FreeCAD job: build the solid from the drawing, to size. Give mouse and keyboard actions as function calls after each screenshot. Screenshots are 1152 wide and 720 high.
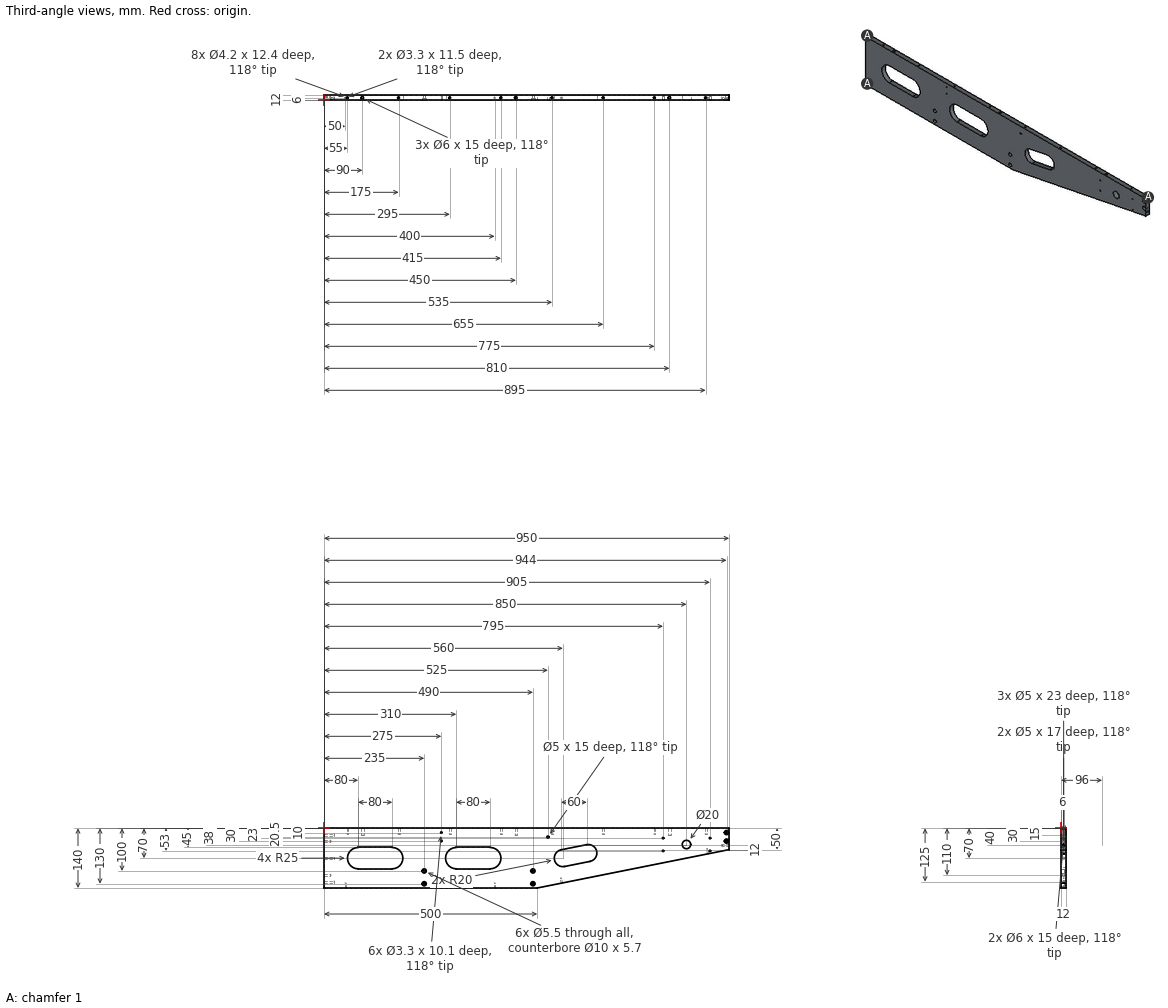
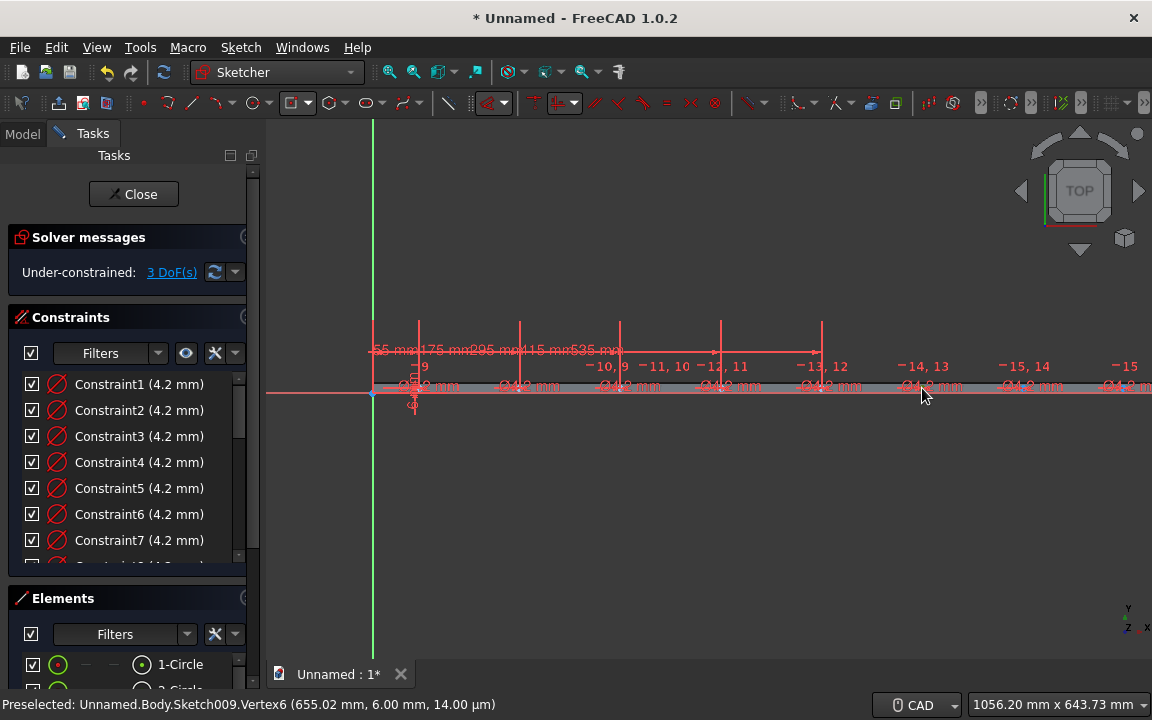
key(l)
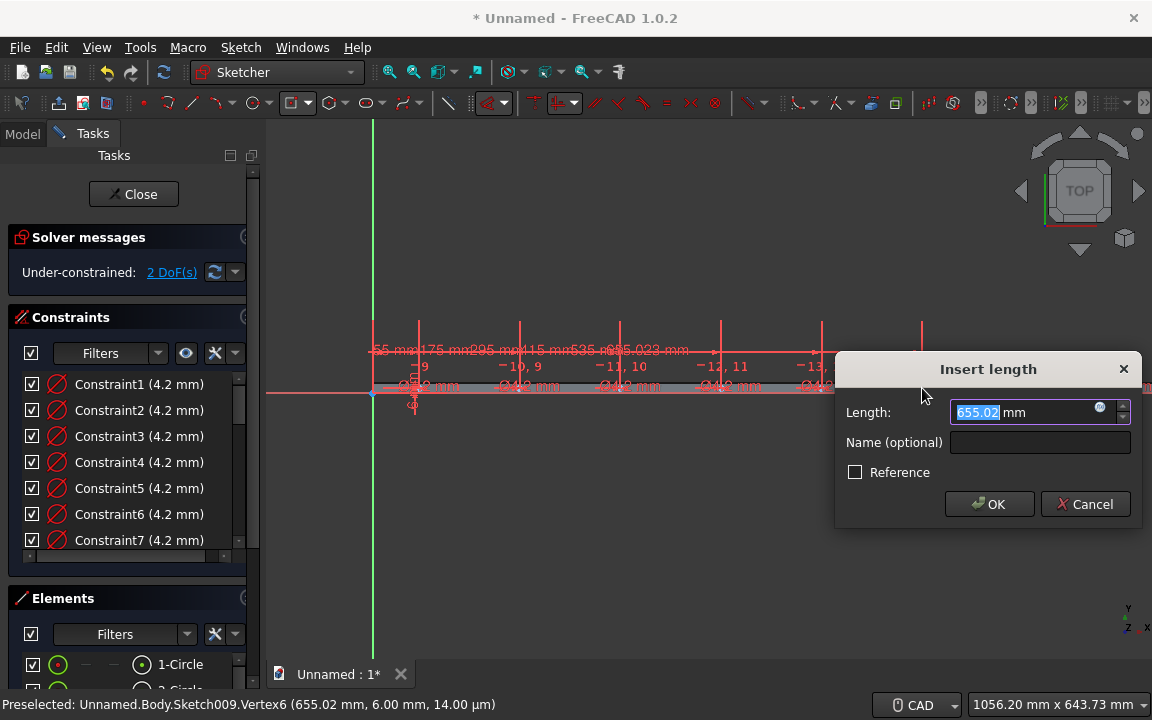
text(655)
key(Return)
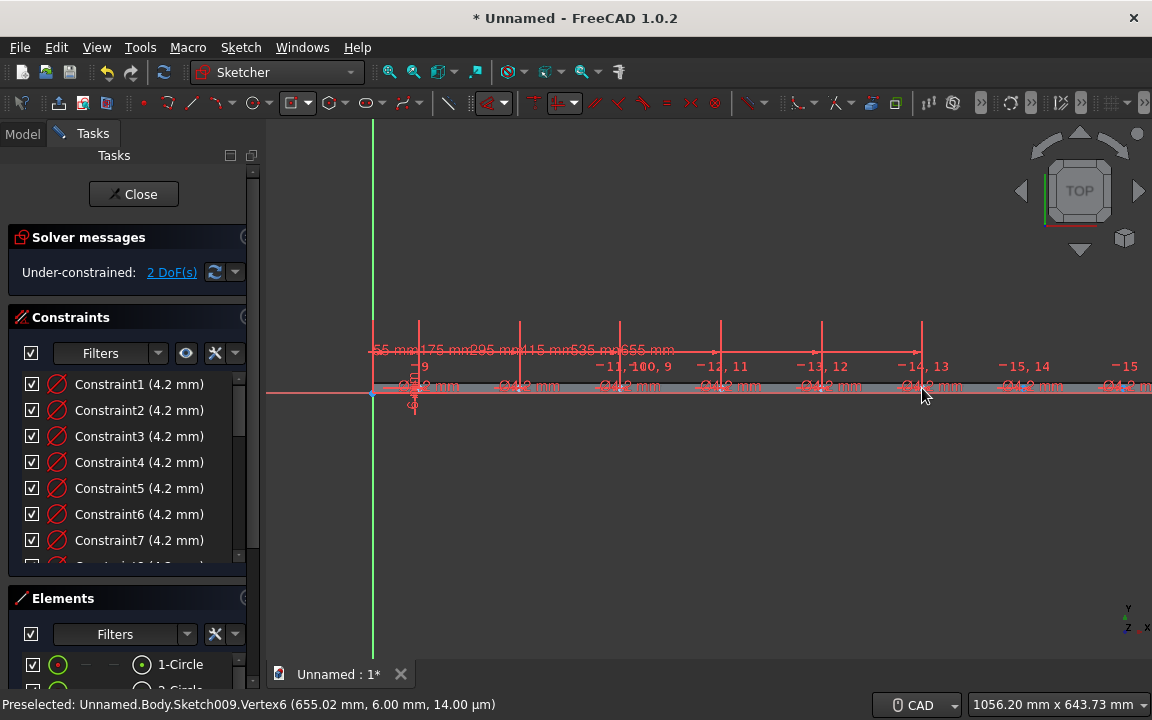
scroll(419, 387, down, 2)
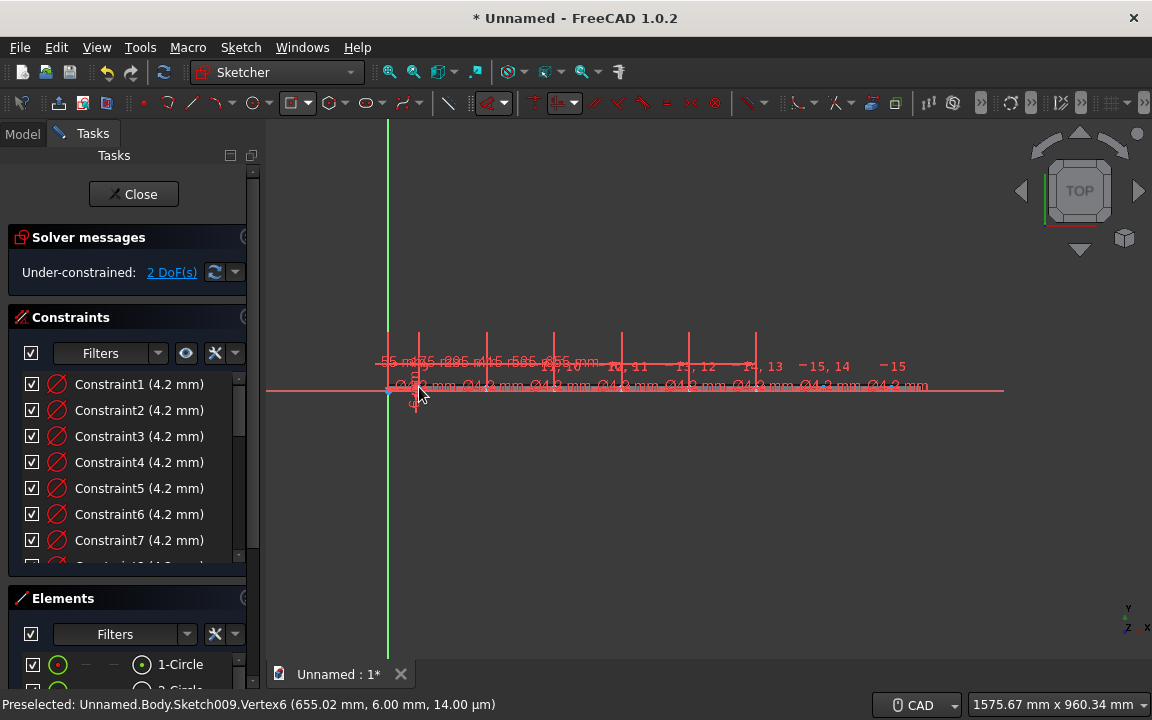
click(824, 388)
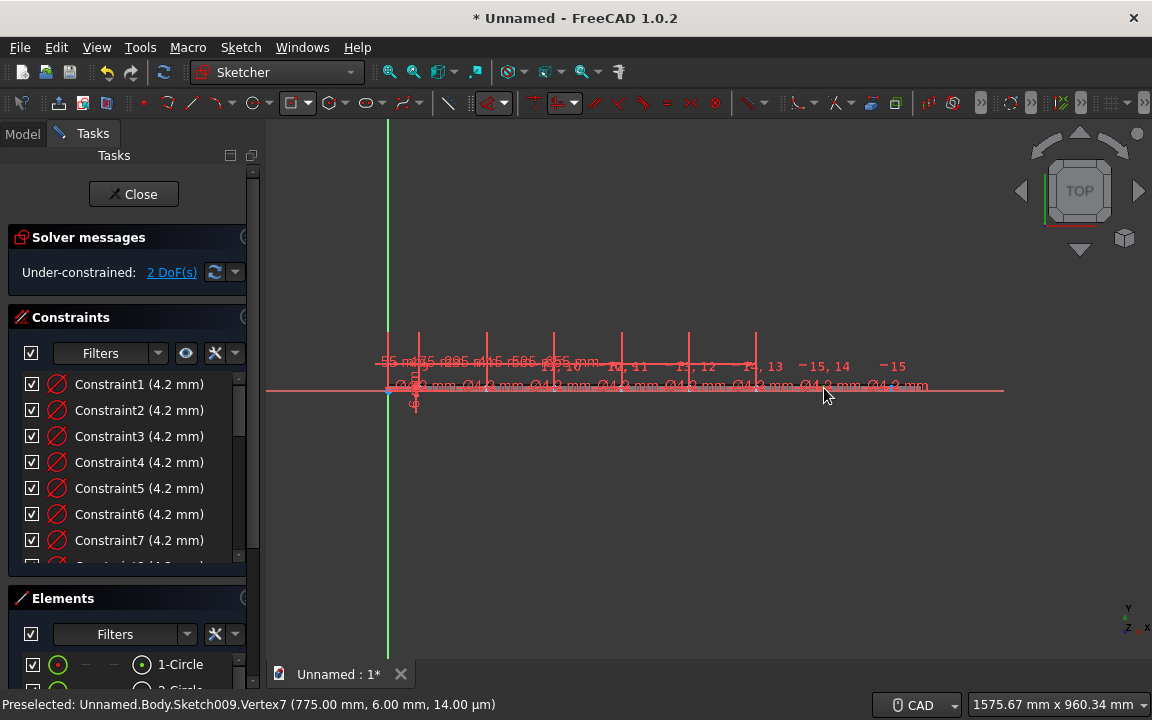
key(l)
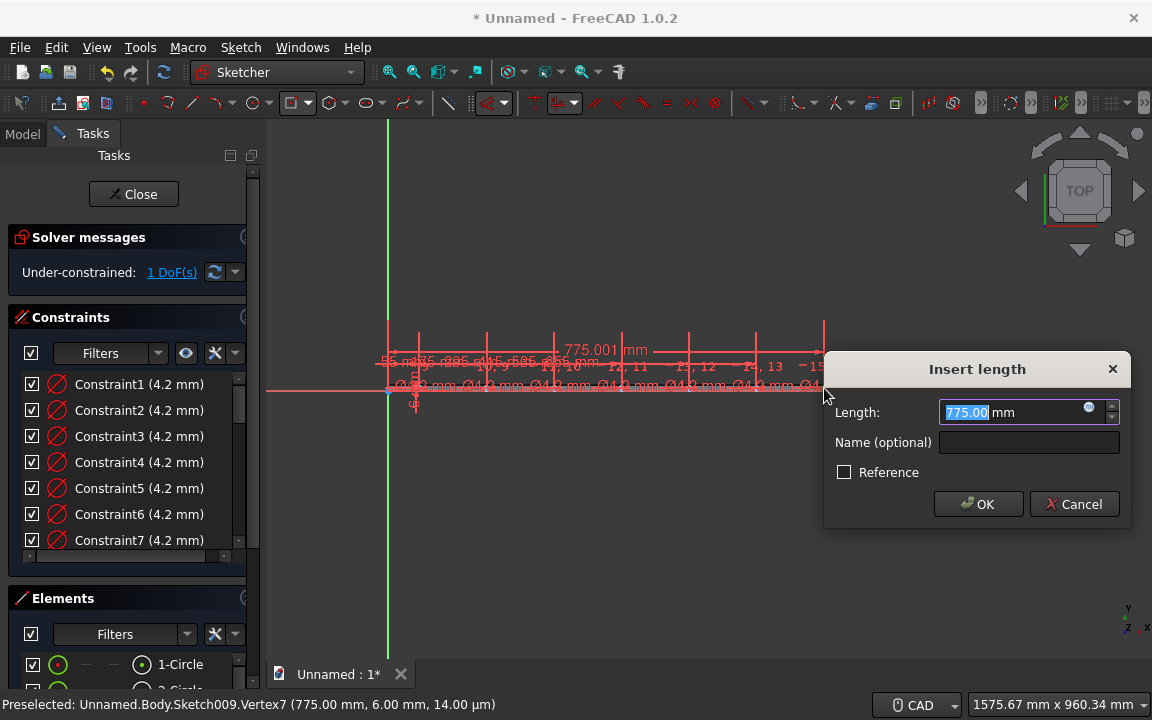
text(775)
key(Return)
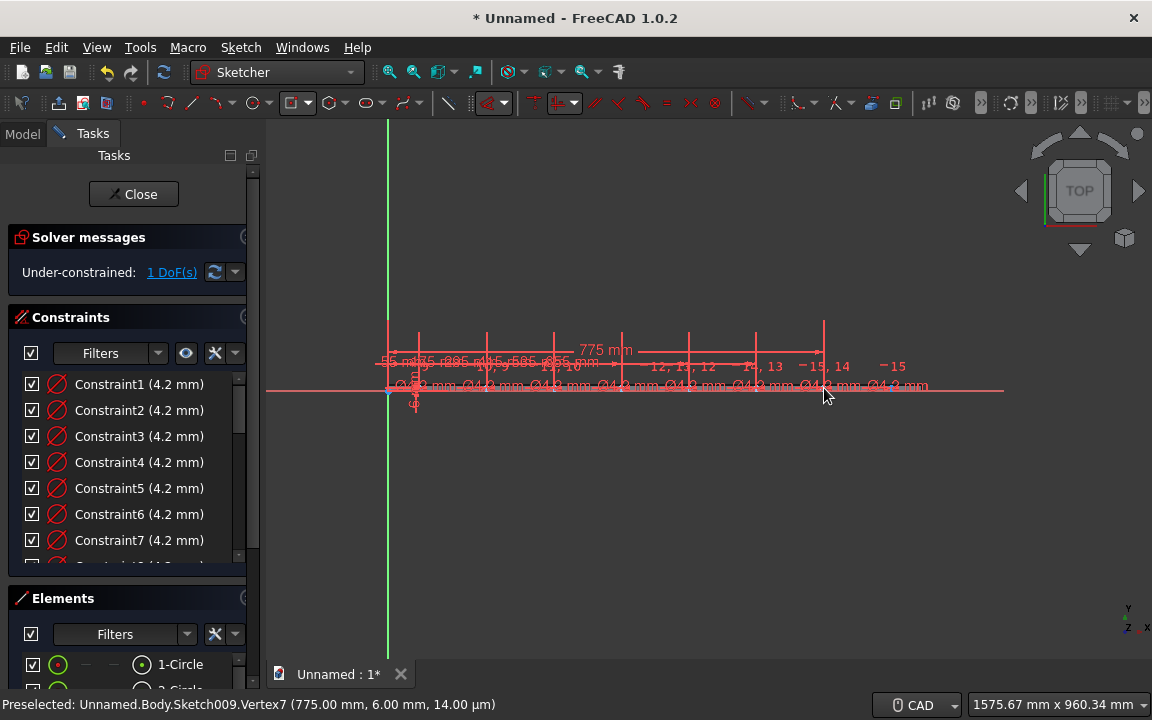
click(891, 388)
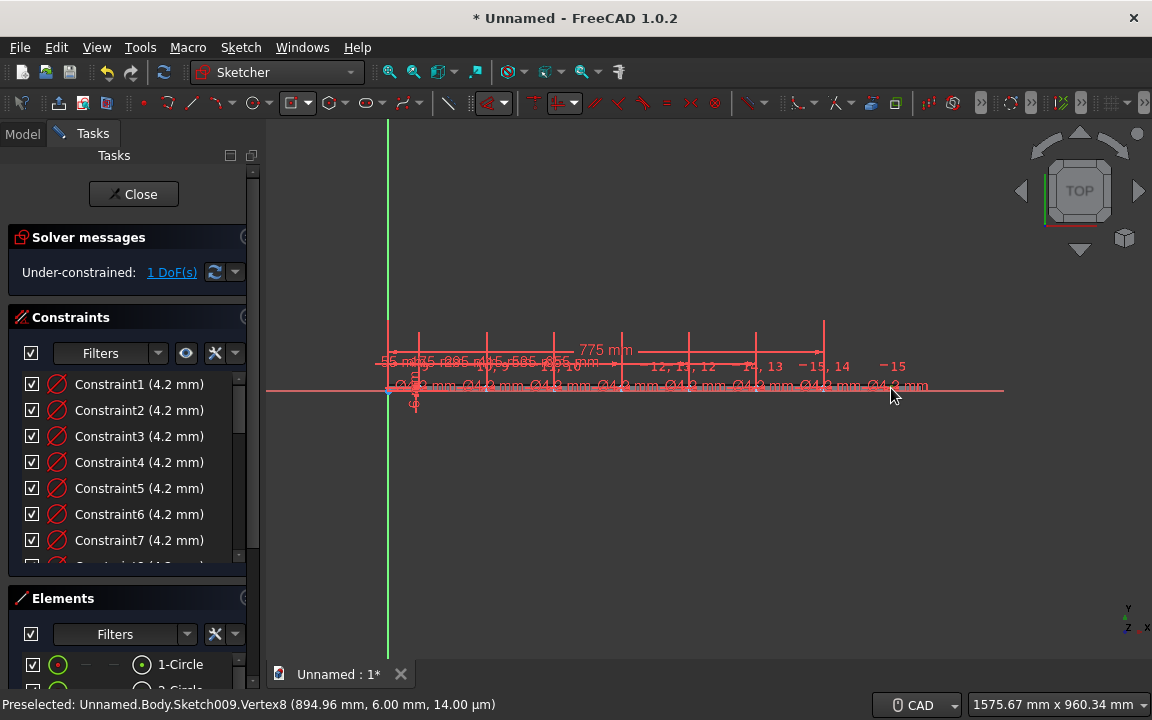
key(l)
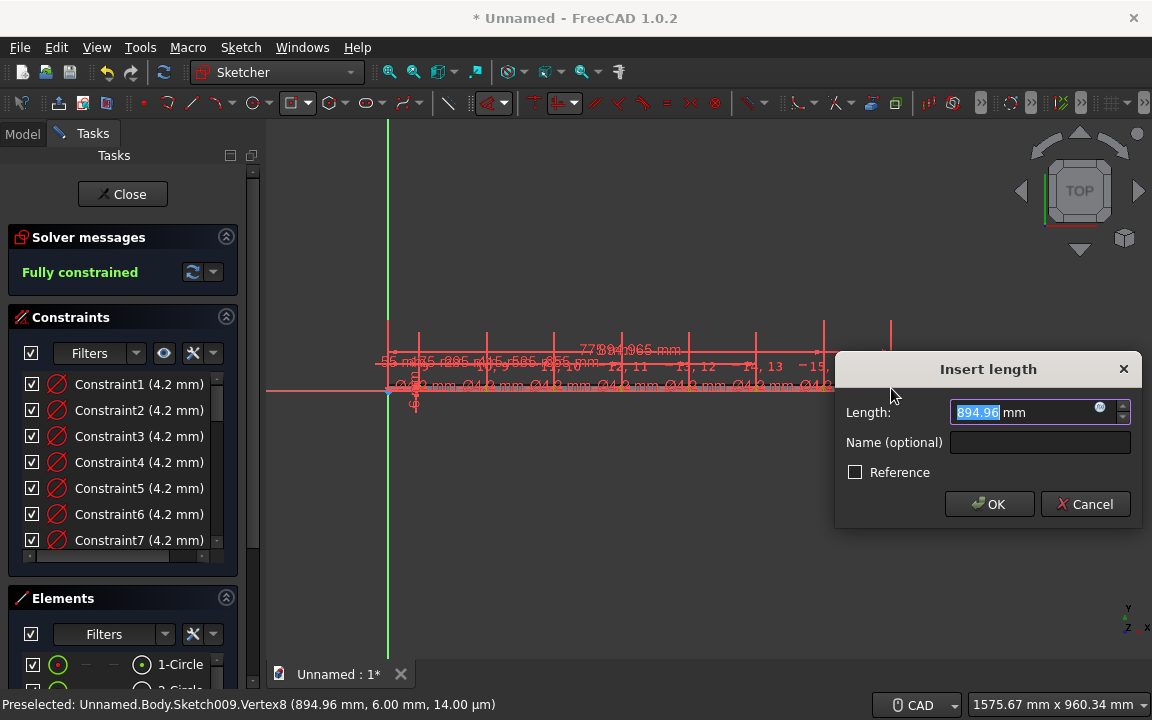
text(895)
key(Return)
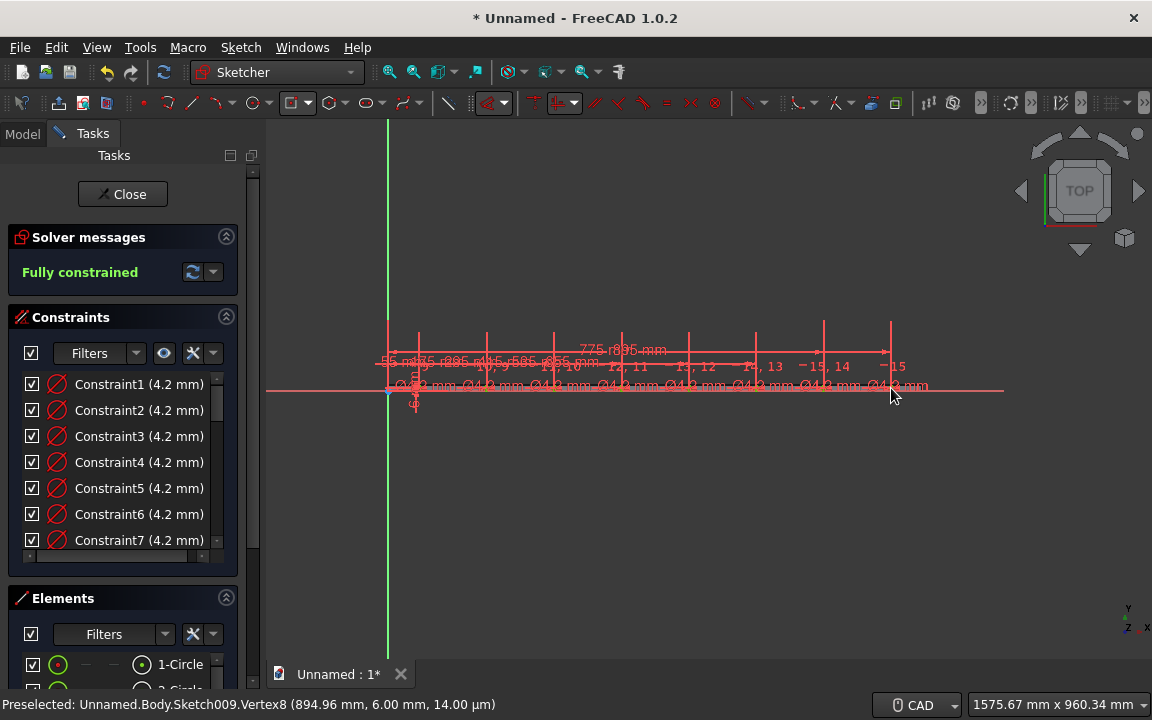
click(123, 194)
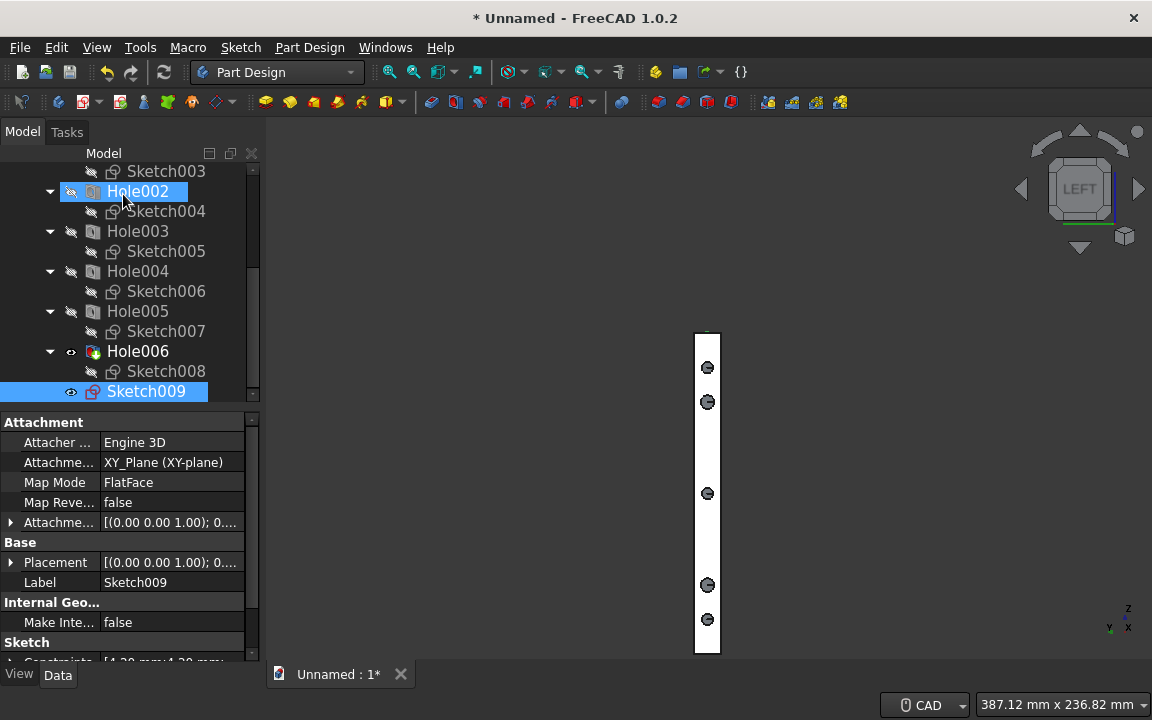
click(456, 102)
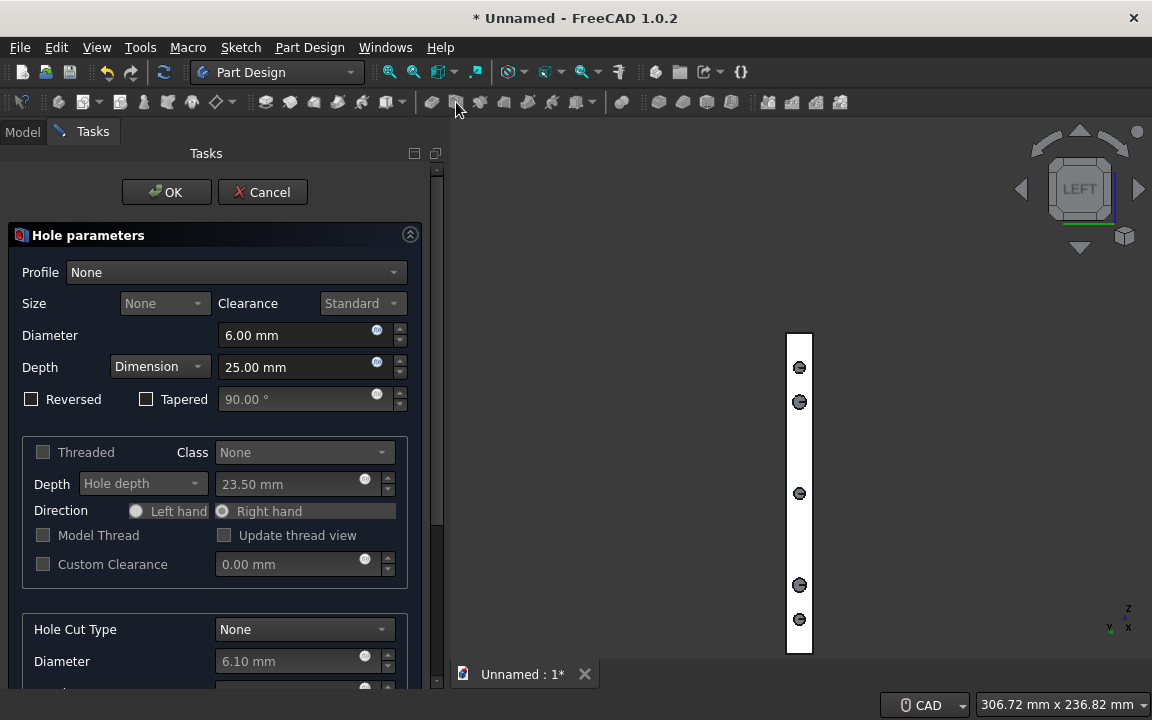
triple_click(305, 335)